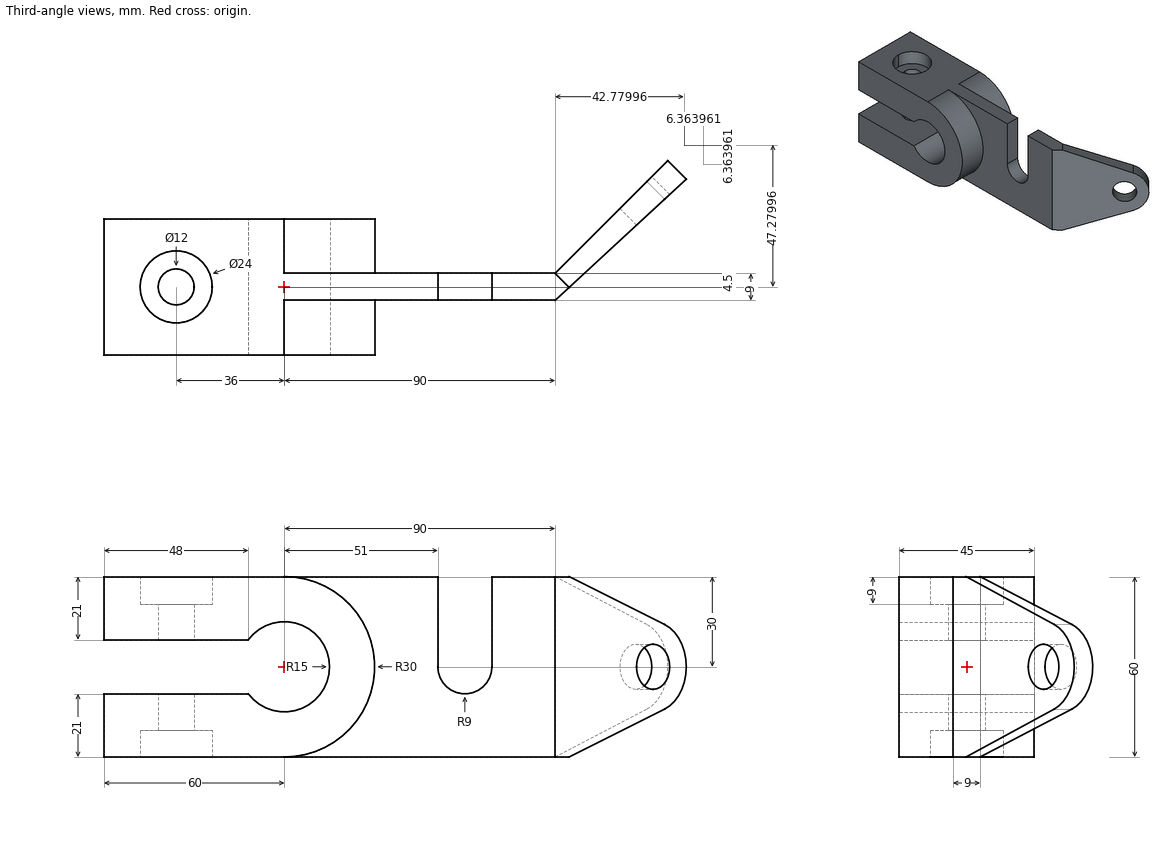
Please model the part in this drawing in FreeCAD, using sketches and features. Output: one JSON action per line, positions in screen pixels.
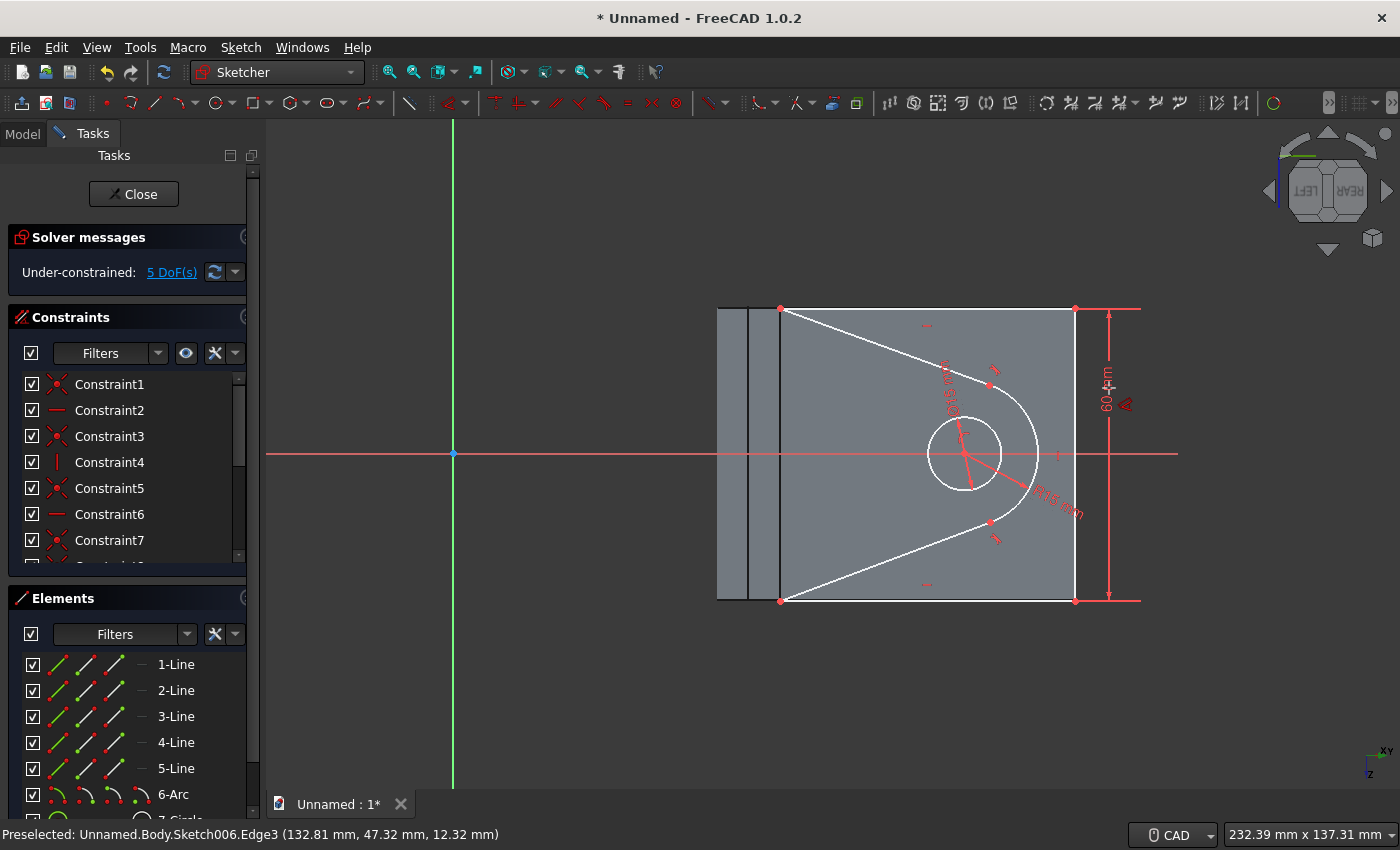
{"action": "left_click", "coordinate": [780, 601]}
{"action": "left_click", "coordinate": [419, 528]}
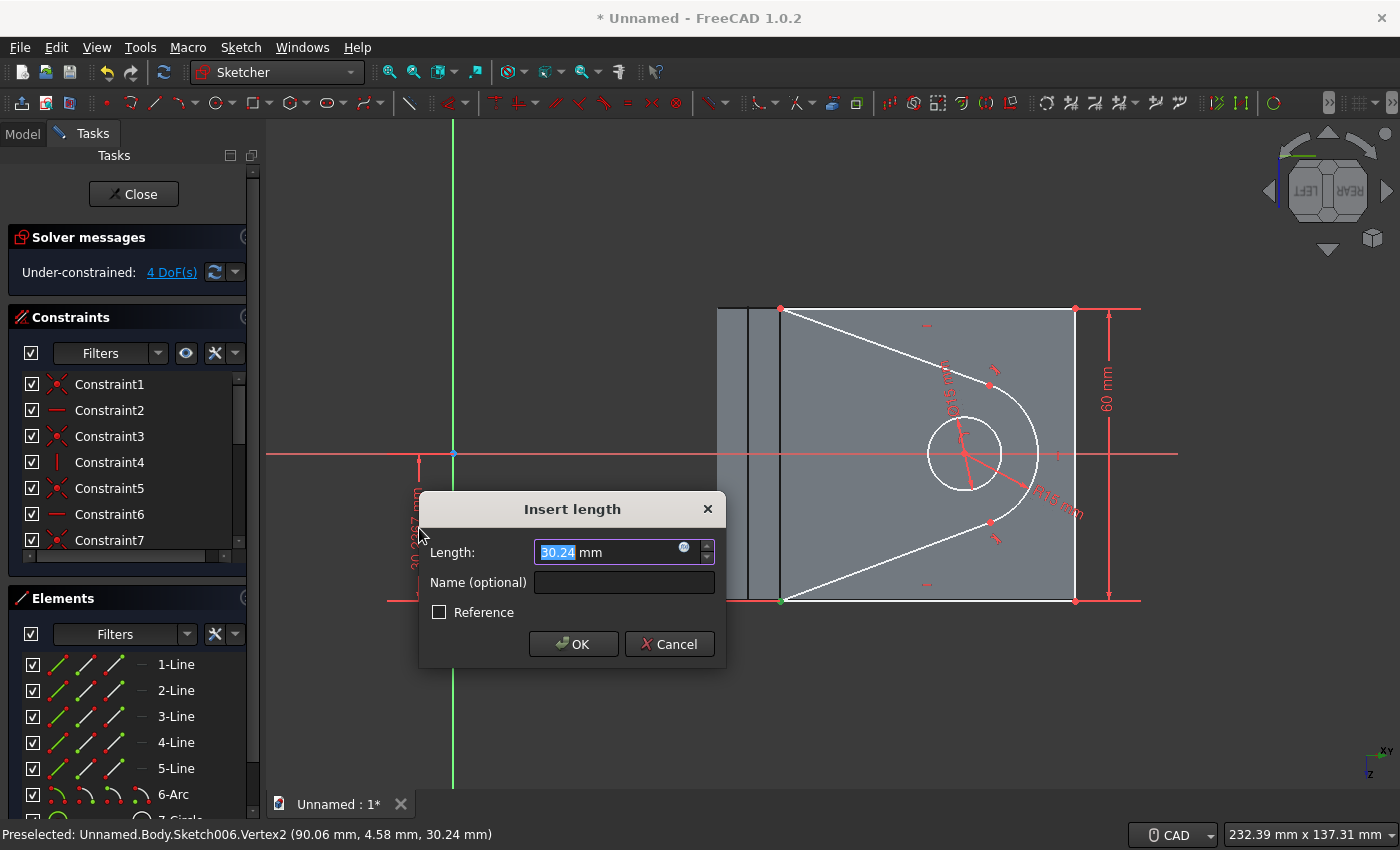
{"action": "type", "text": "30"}
{"action": "key", "text": "Return"}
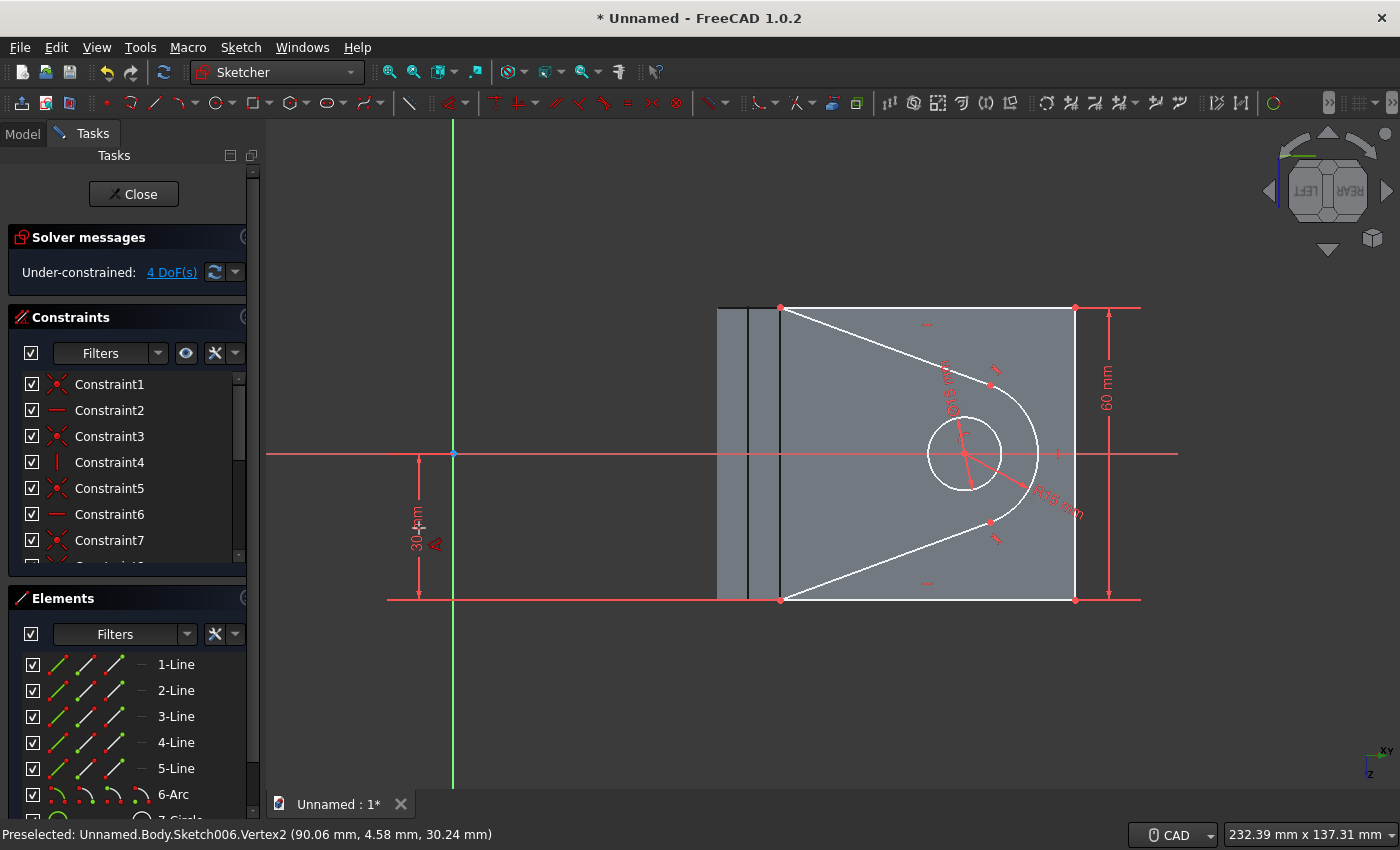
{"action": "left_click", "coordinate": [868, 600]}
{"action": "left_click", "coordinate": [927, 634]}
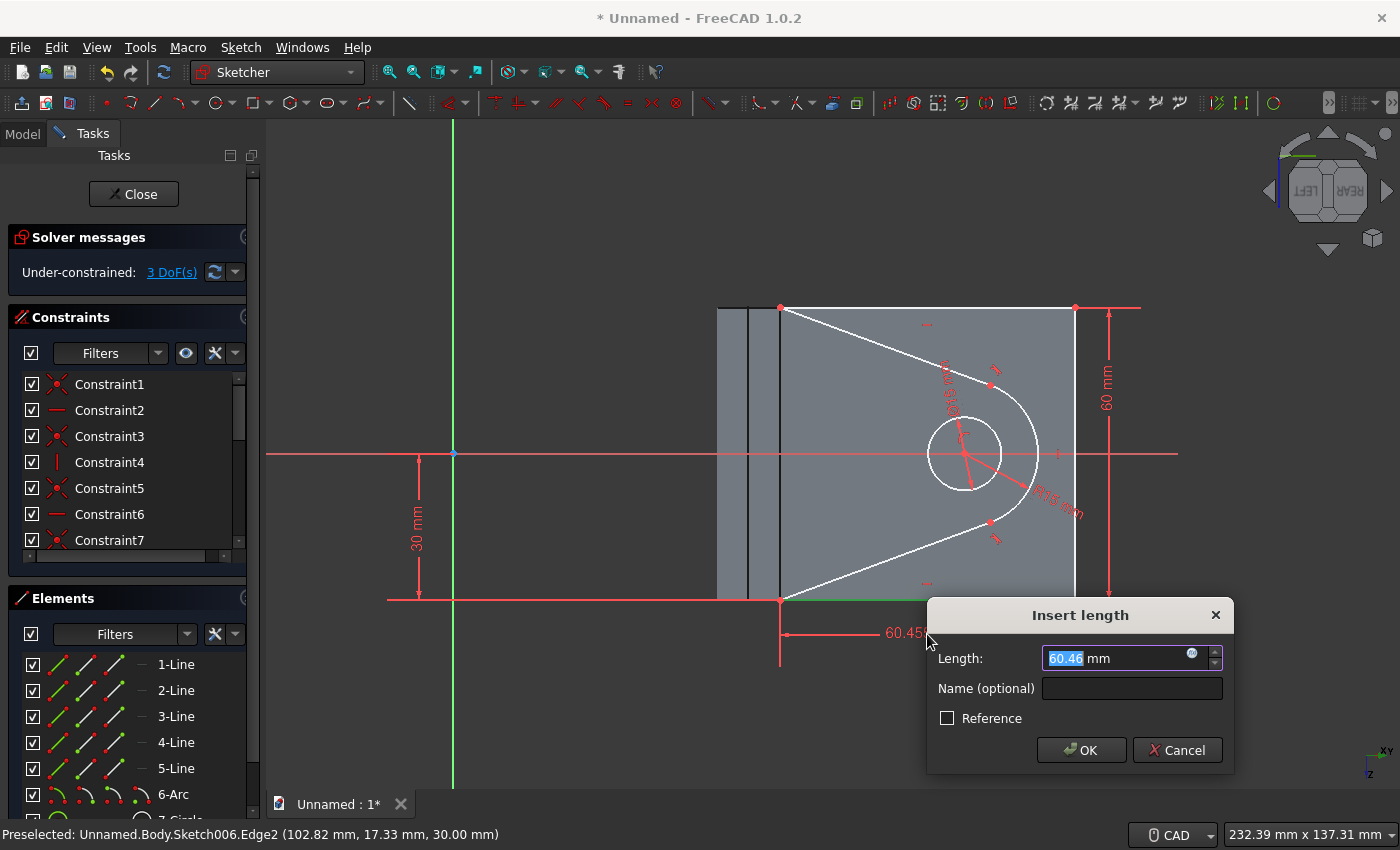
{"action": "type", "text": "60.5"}
{"action": "key", "text": "Return"}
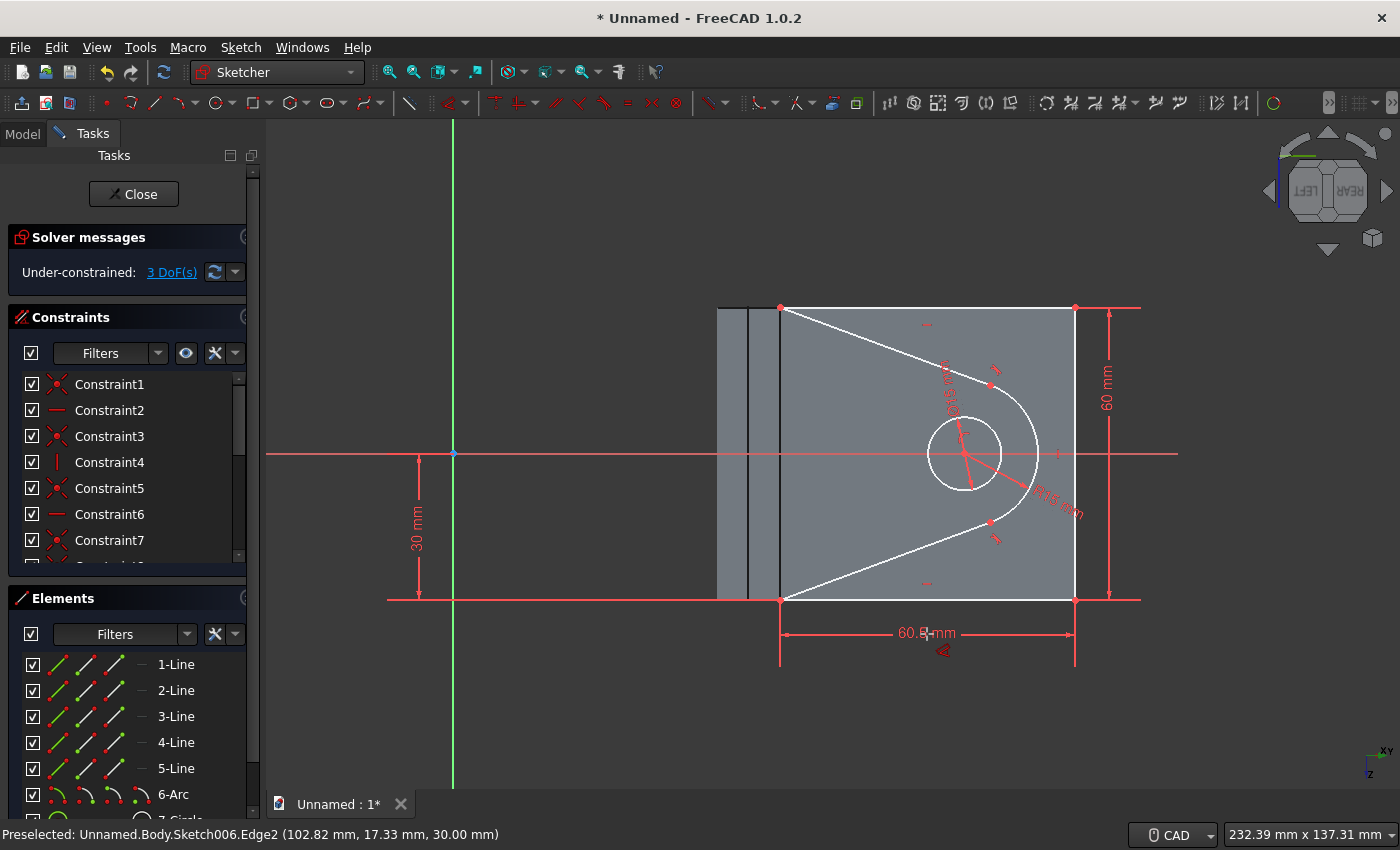
{"action": "left_click", "coordinate": [987, 308]}
{"action": "left_click", "coordinate": [928, 274]}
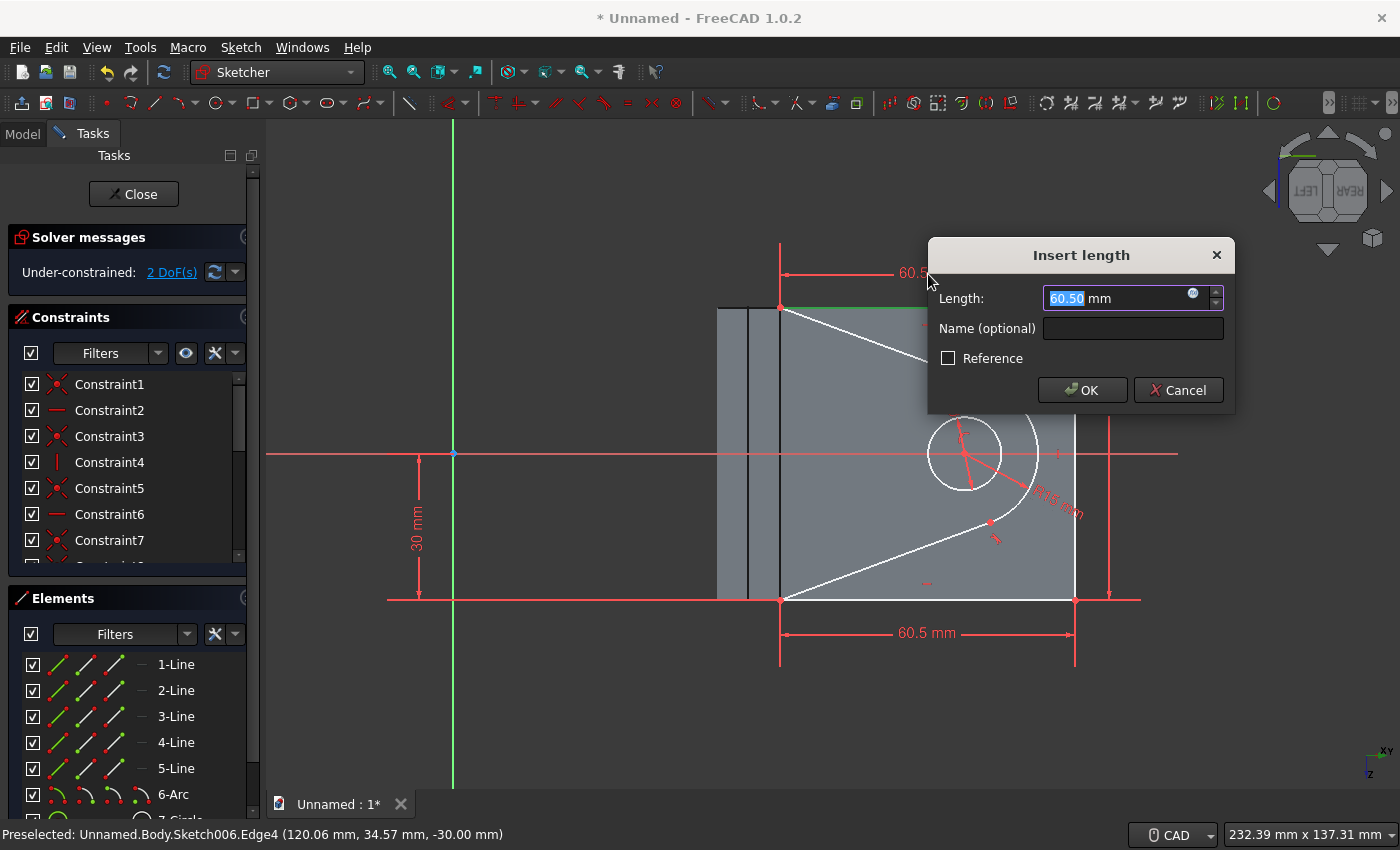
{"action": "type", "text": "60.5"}
{"action": "key", "text": "Return"}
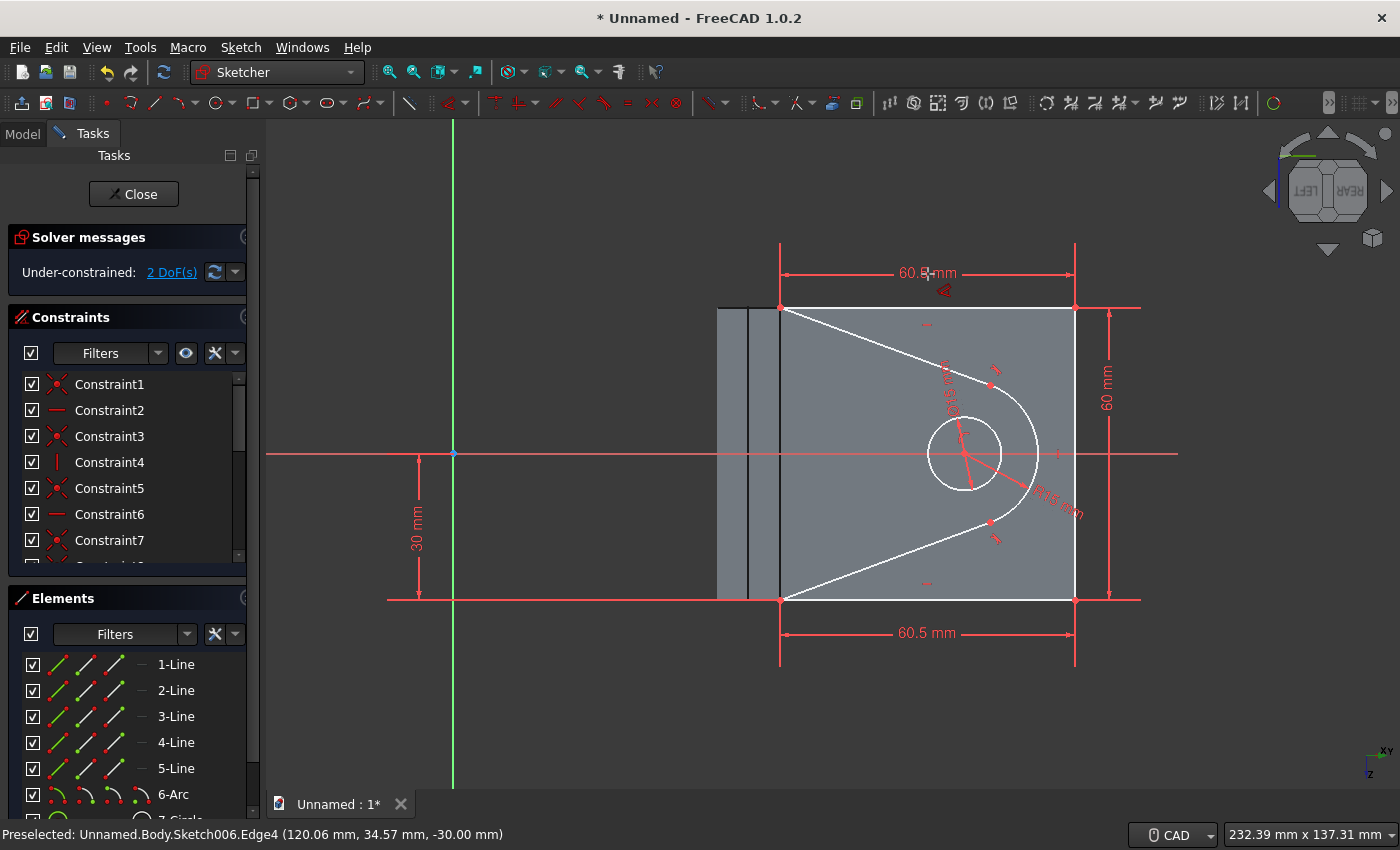
{"action": "left_click", "coordinate": [1075, 600]}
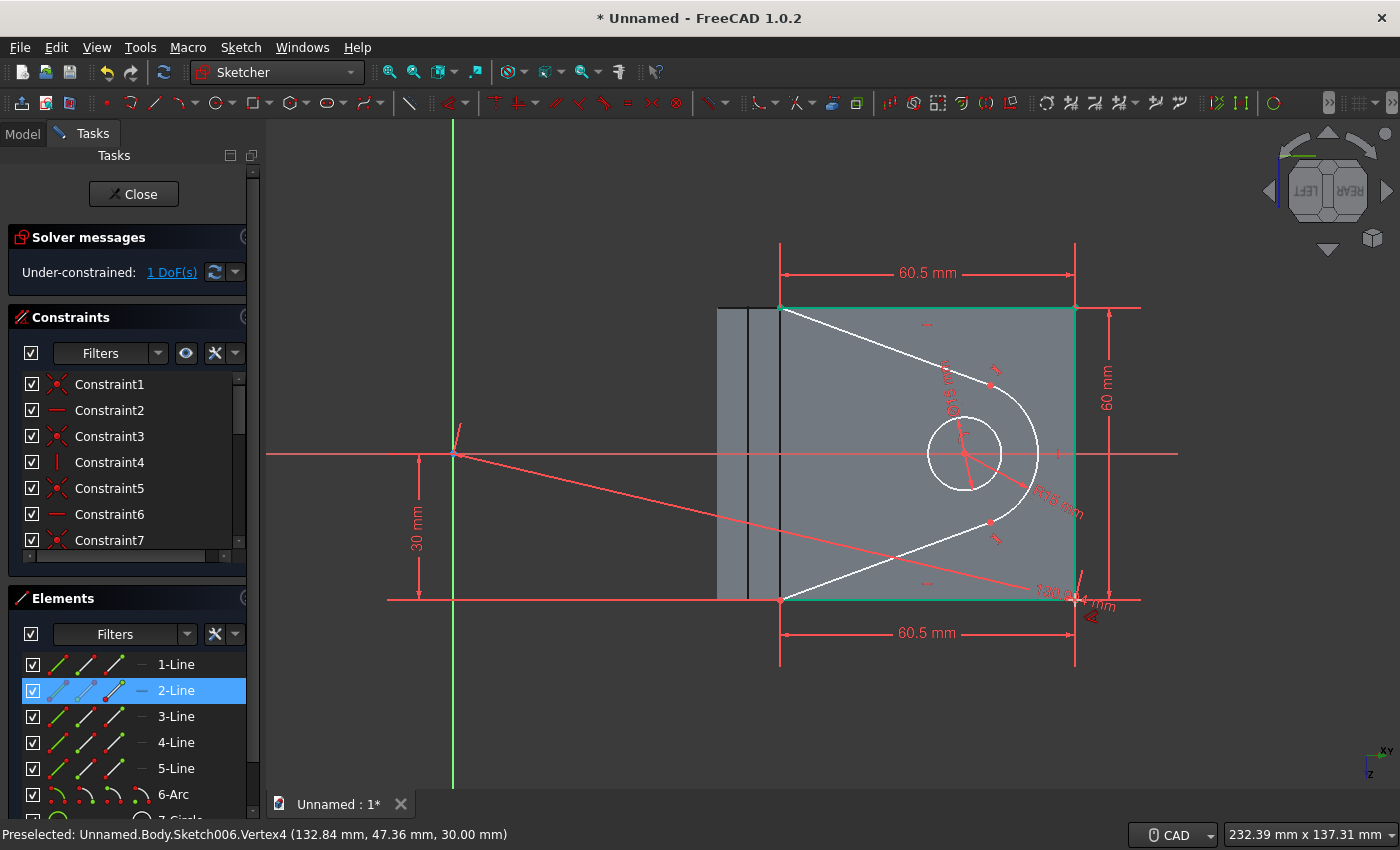
{"action": "left_click", "coordinate": [965, 454]}
{"action": "left_click", "coordinate": [1020, 634]}